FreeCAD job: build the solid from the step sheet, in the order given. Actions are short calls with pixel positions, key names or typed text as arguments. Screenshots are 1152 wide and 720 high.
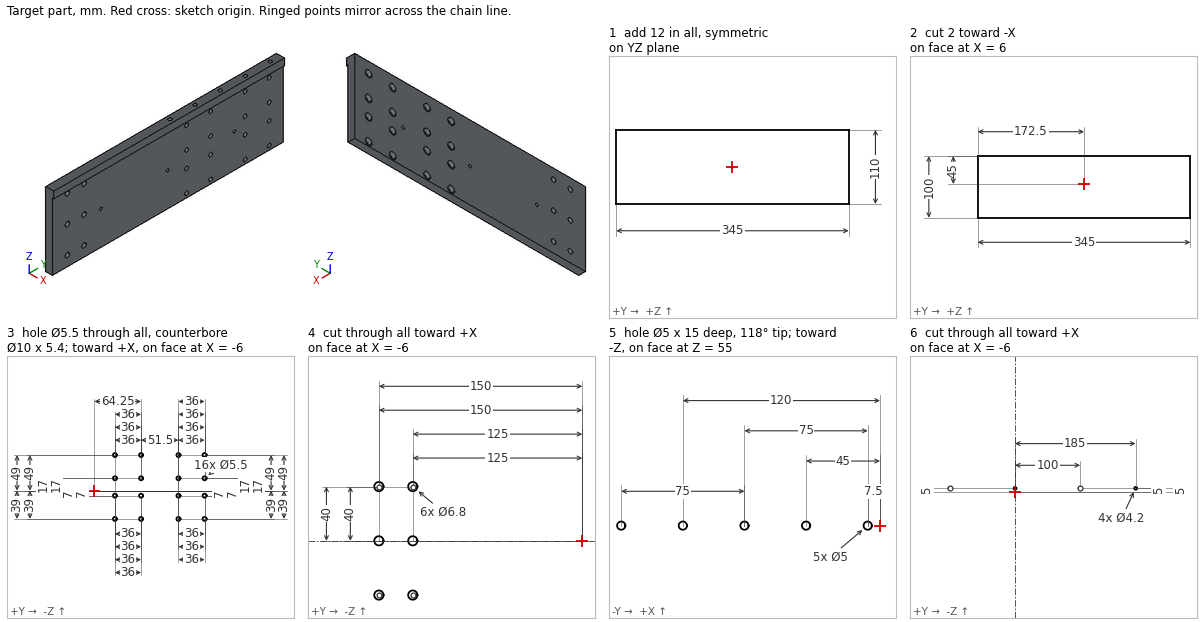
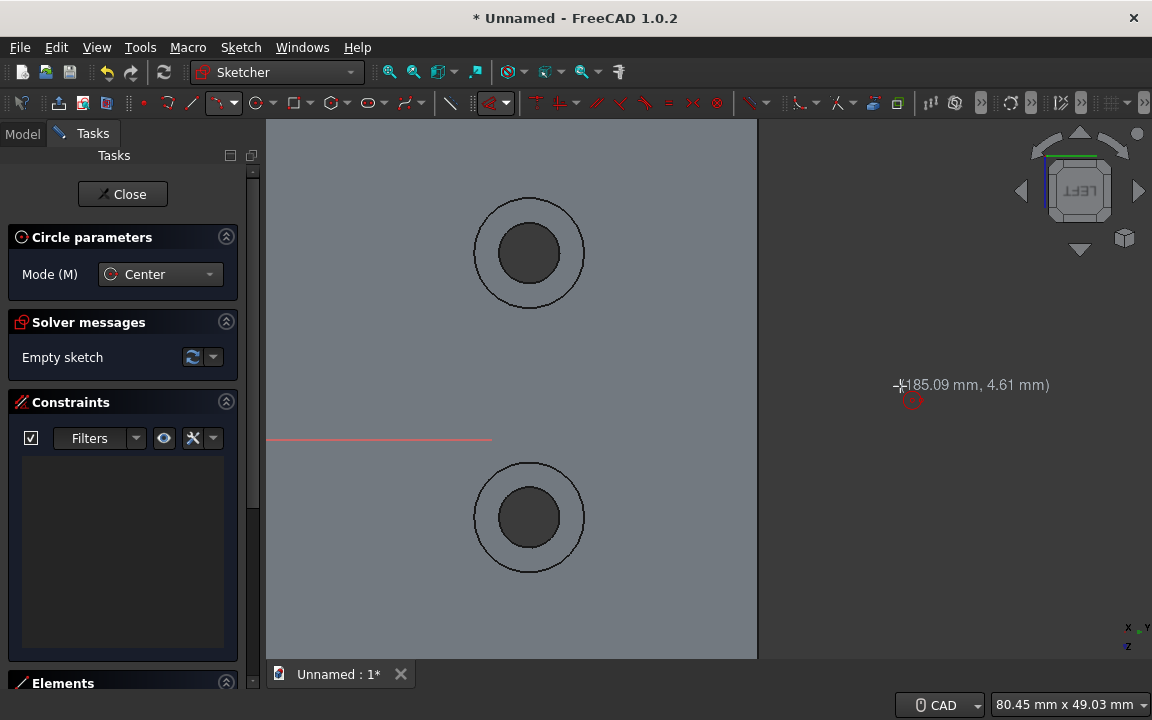
scroll(901, 387, down, 9)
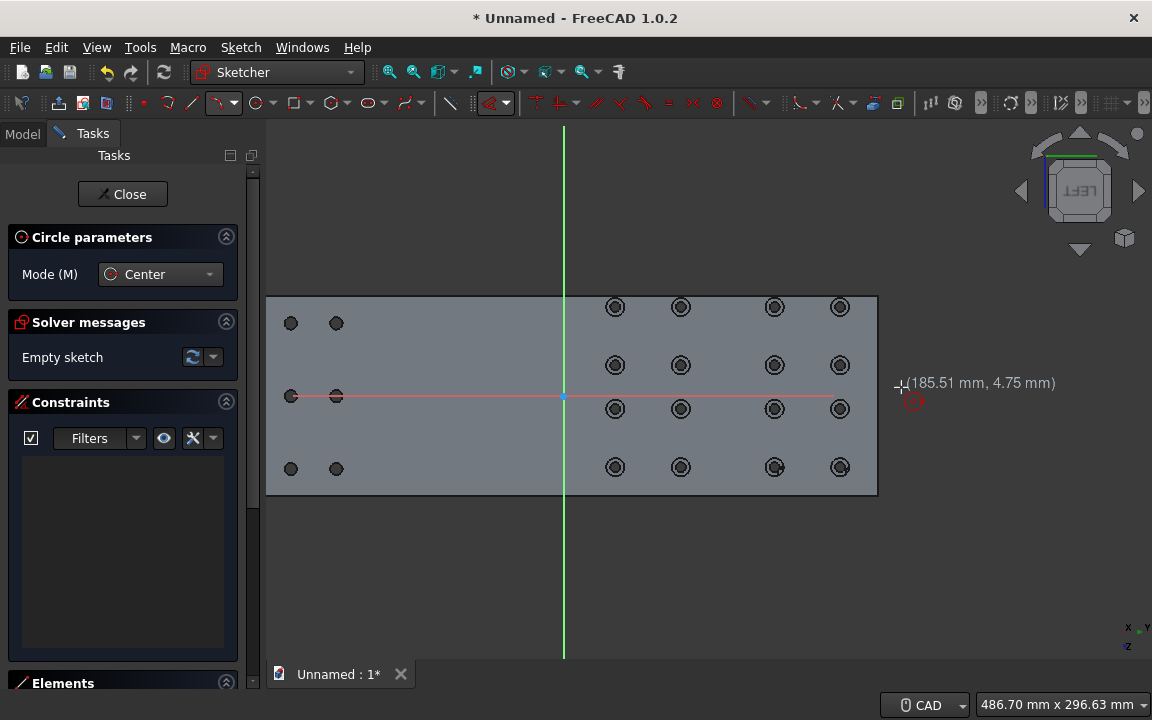
scroll(901, 387, up, 3)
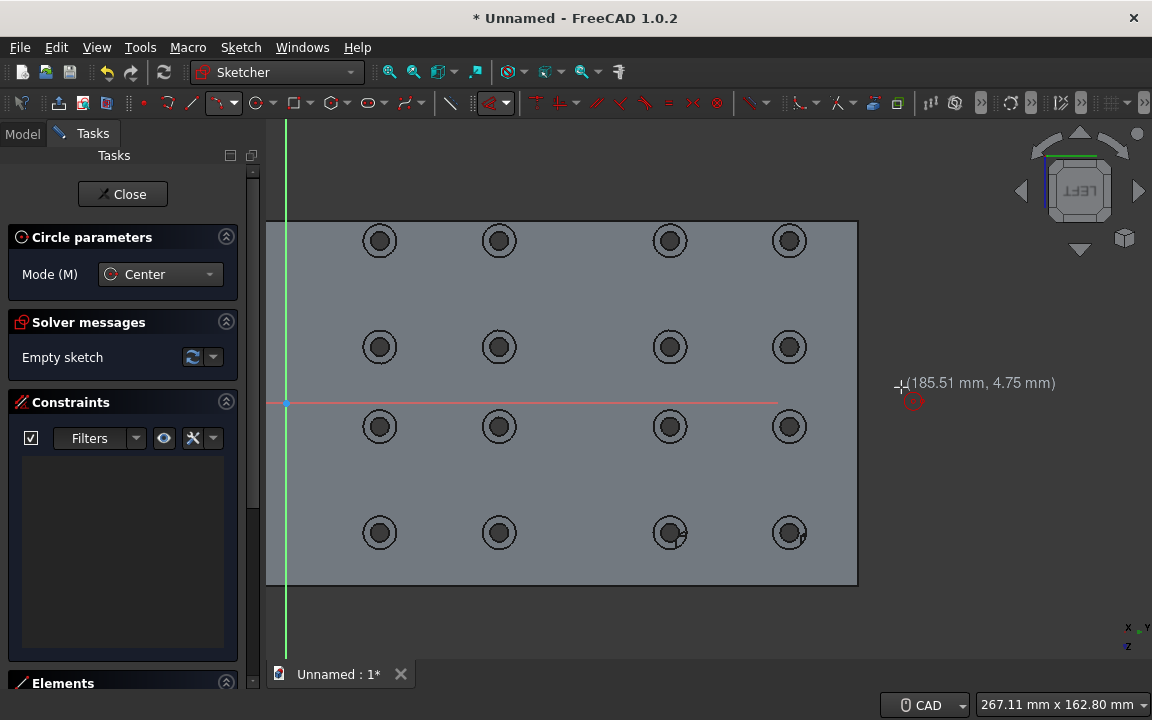
click(900, 387)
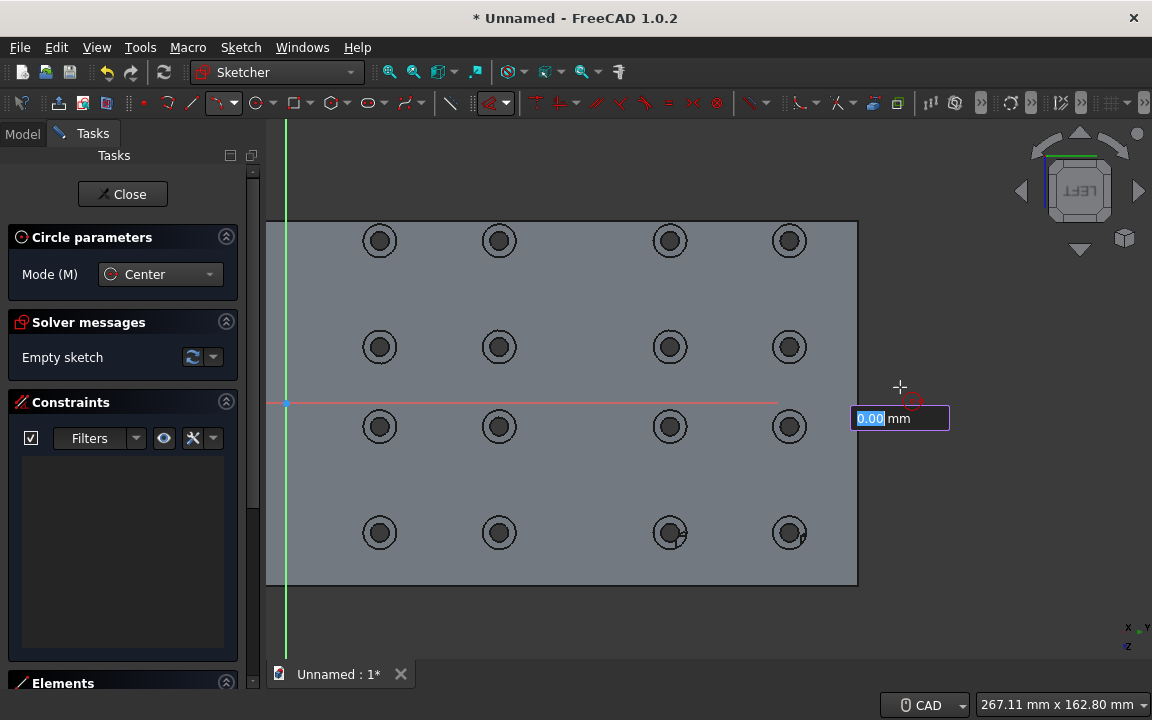
scroll(905, 382, up, 5)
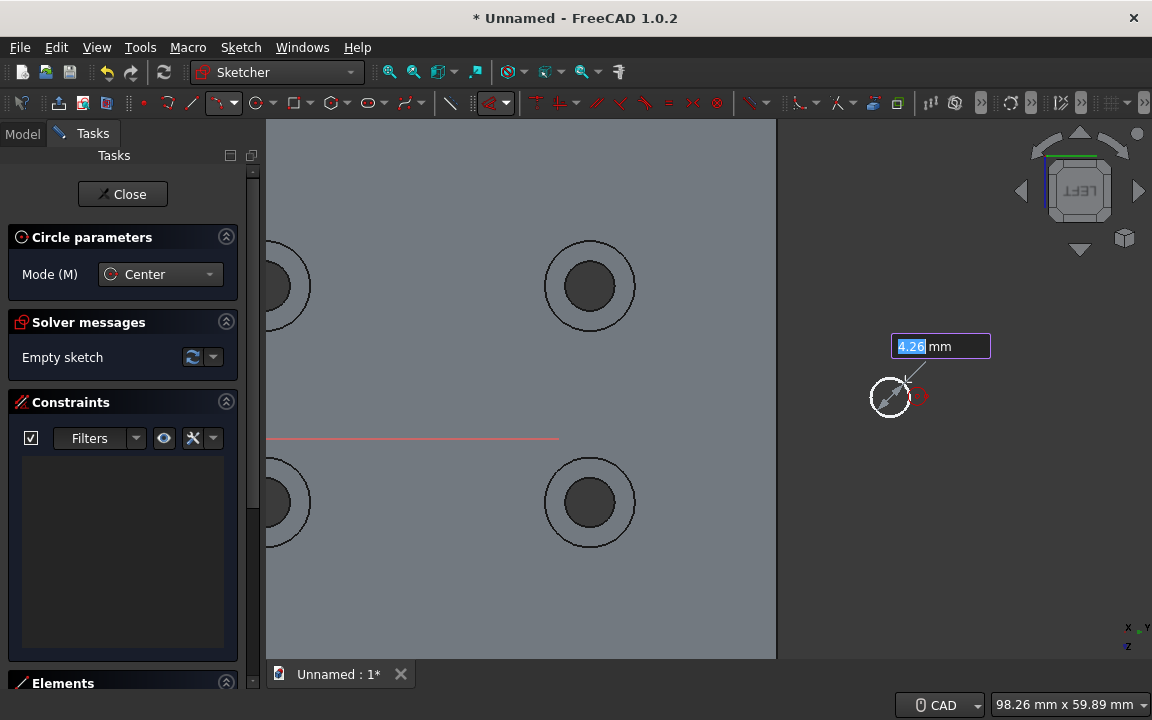
click(903, 381)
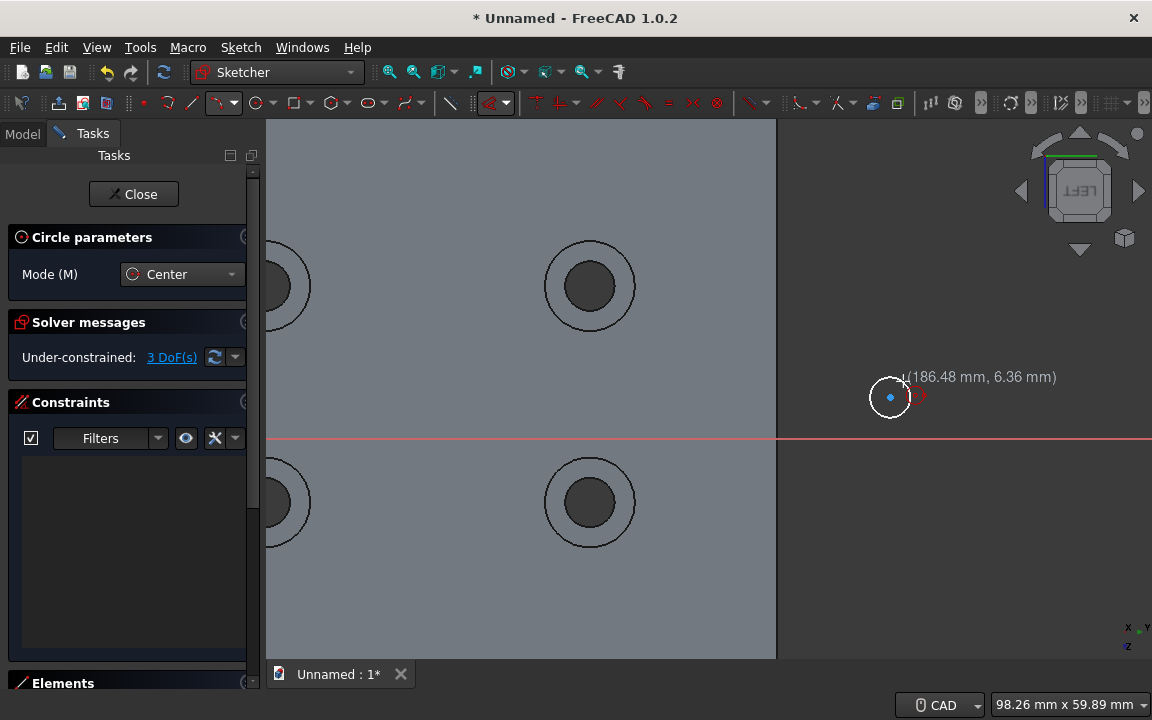
scroll(903, 384, down, 8)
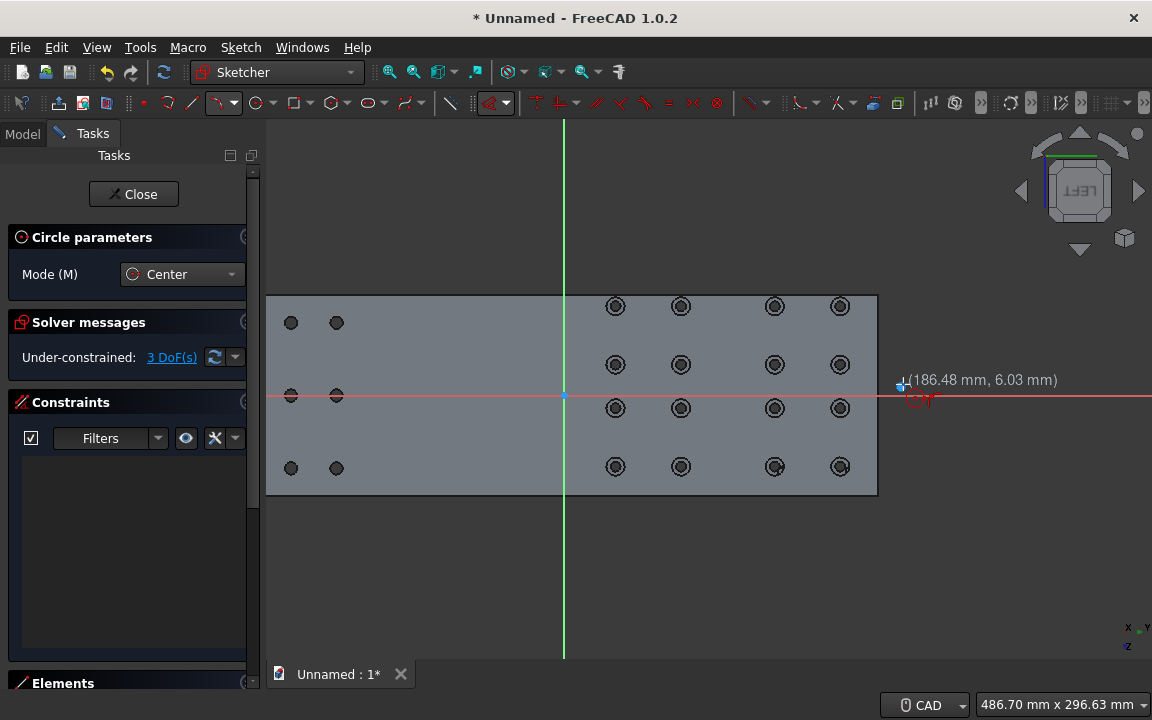
scroll(746, 386, up, 9)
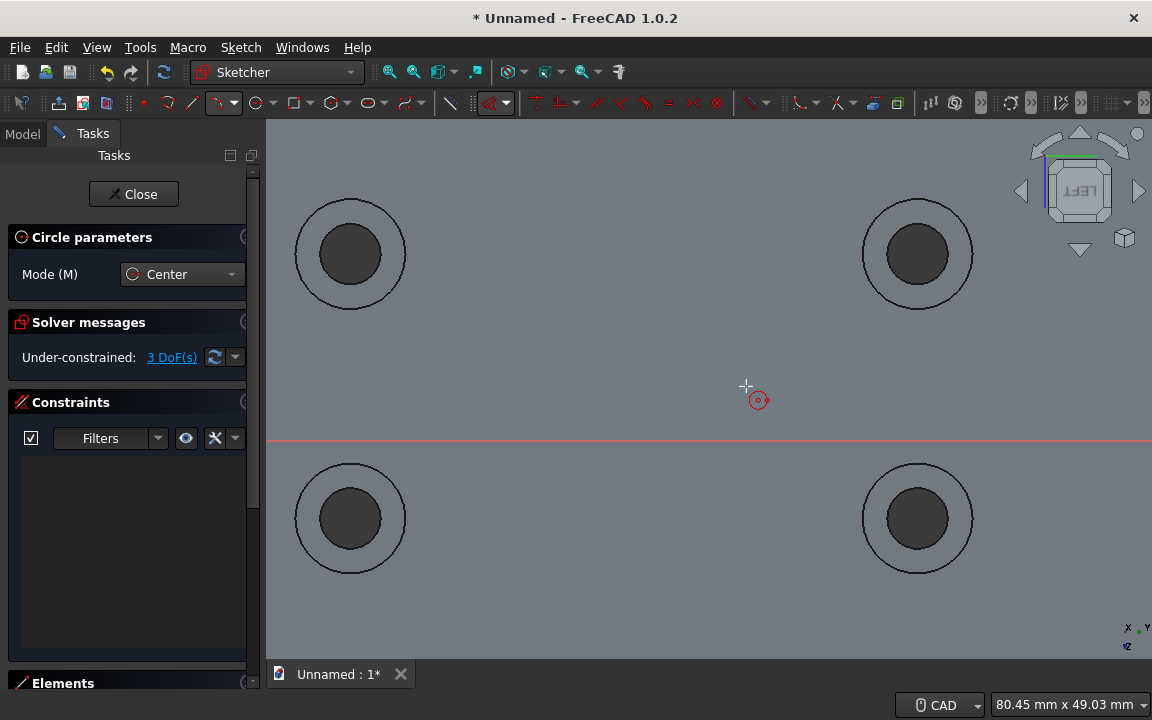
scroll(745, 386, down, 9)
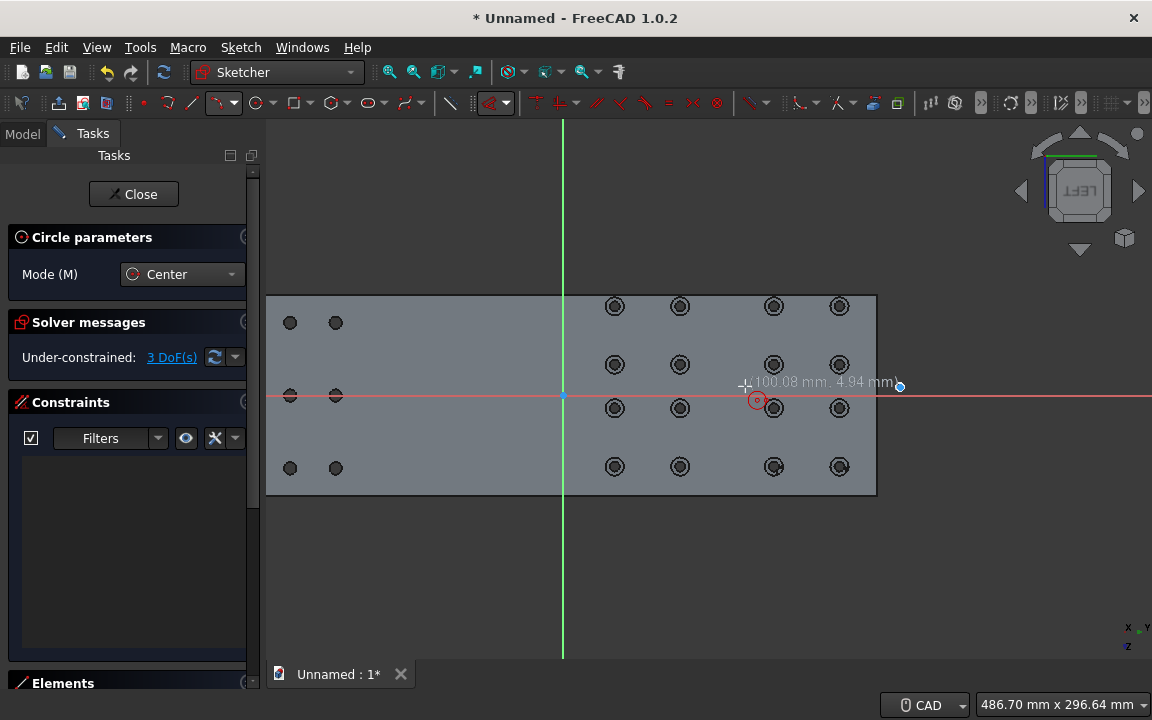
scroll(745, 386, up, 3)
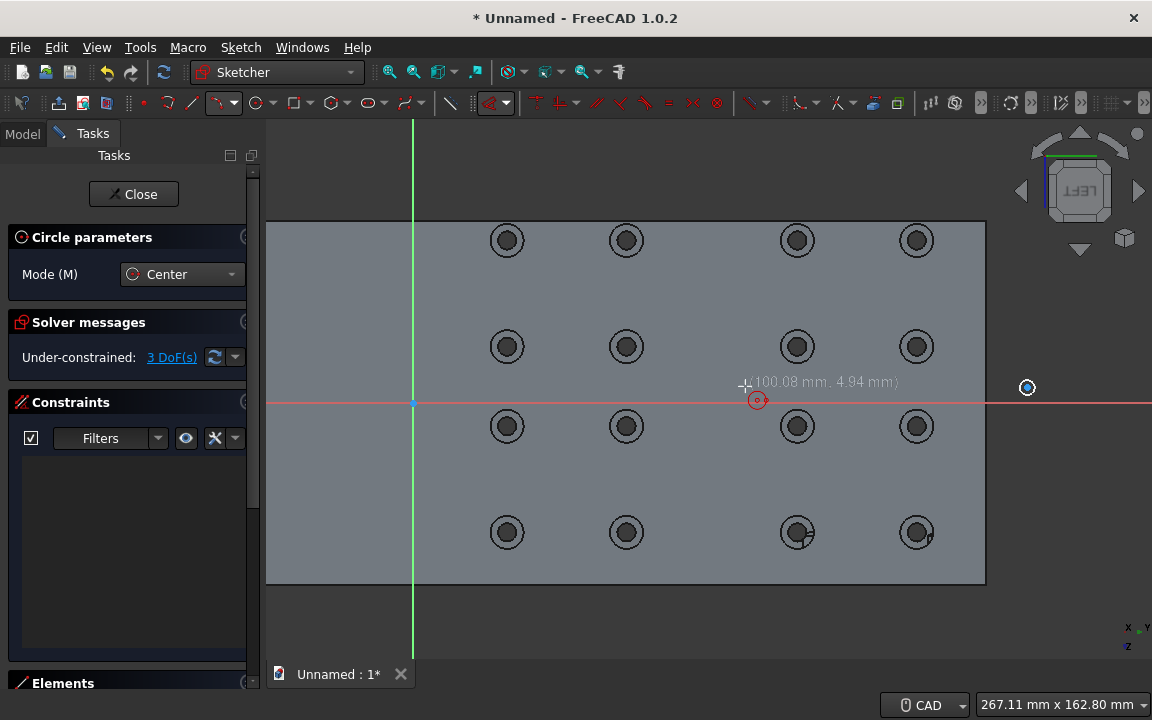
click(745, 386)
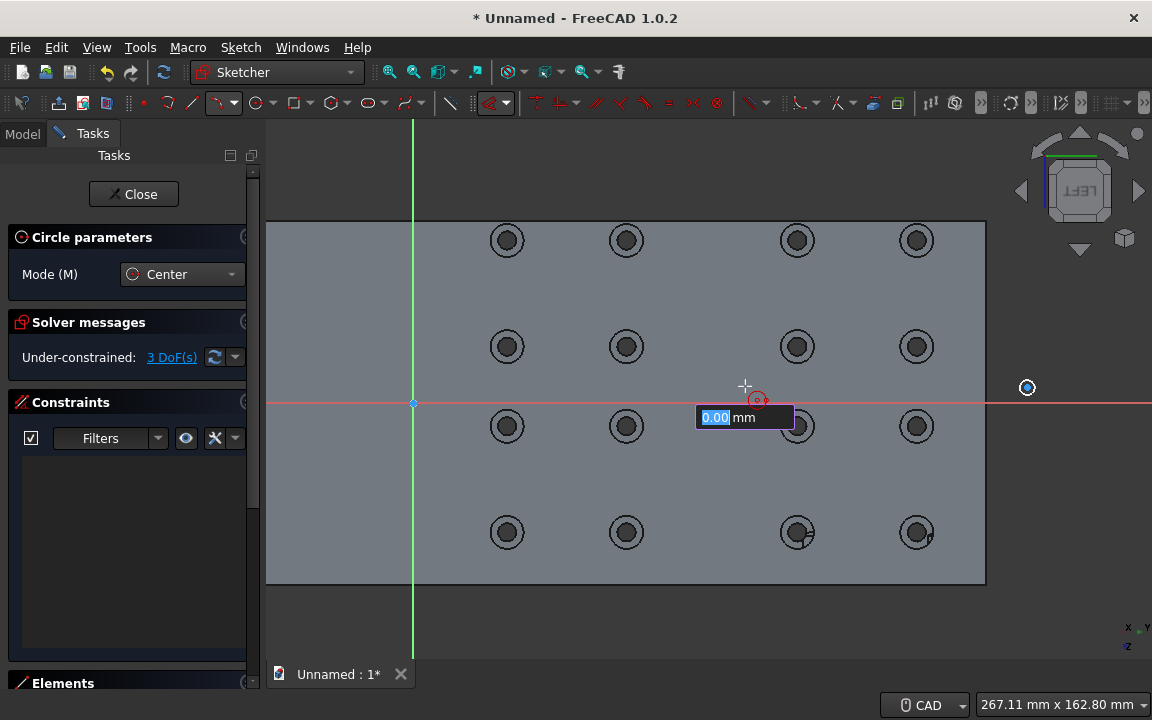
scroll(750, 382, up, 5)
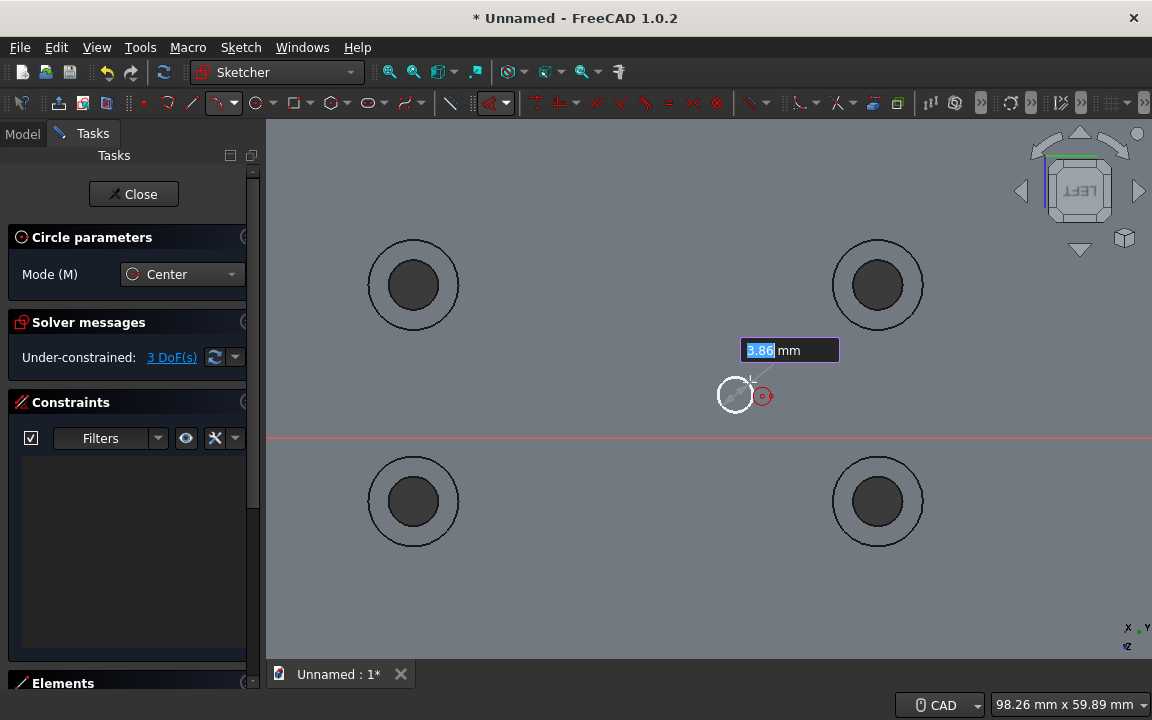
click(749, 380)